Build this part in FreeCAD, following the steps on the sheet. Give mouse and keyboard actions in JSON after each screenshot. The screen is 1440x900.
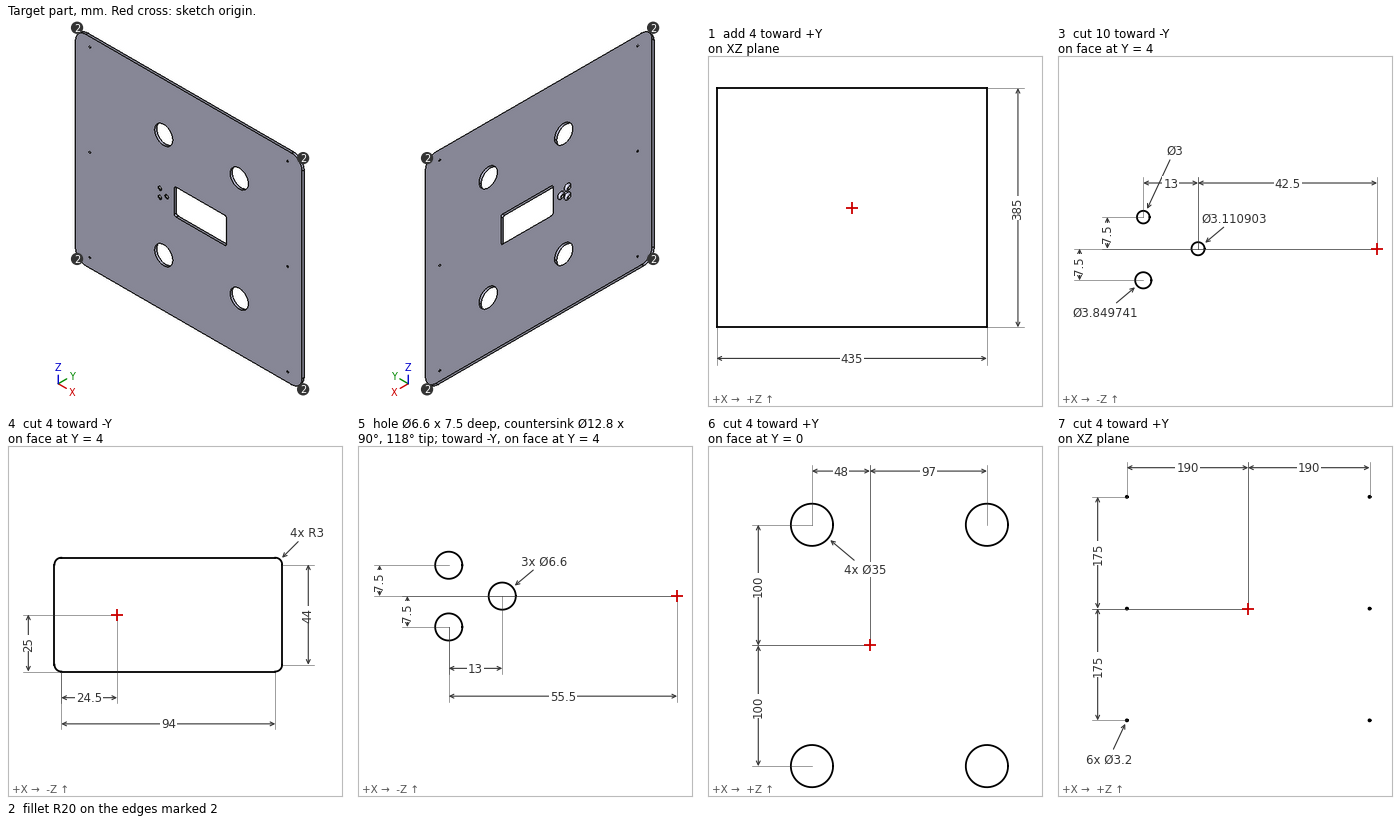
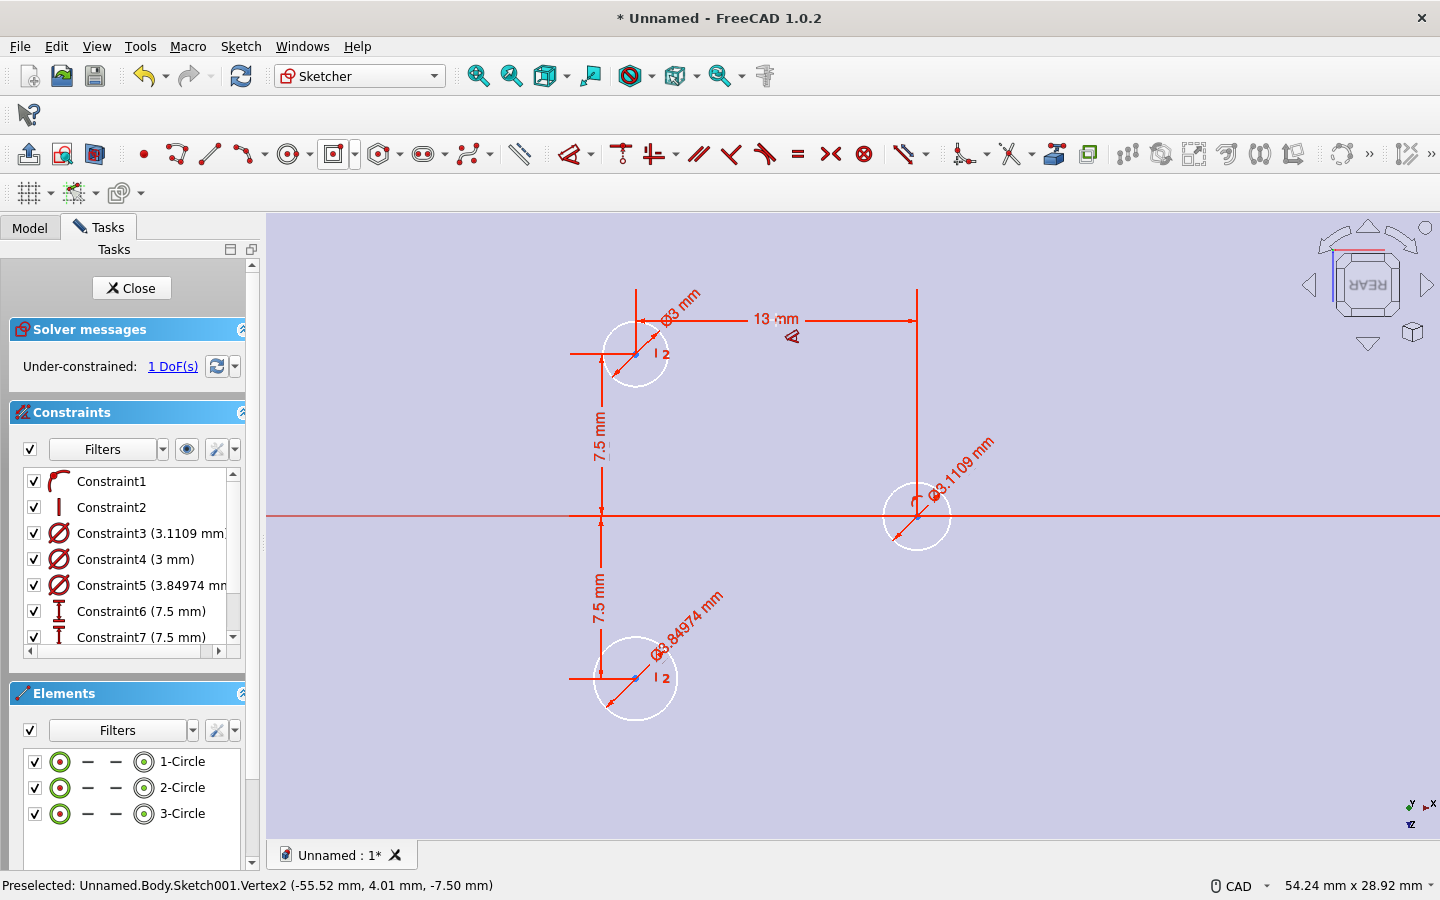
{"action": "left_click", "coordinate": [917, 516]}
{"action": "left_click", "coordinate": [1096, 482]}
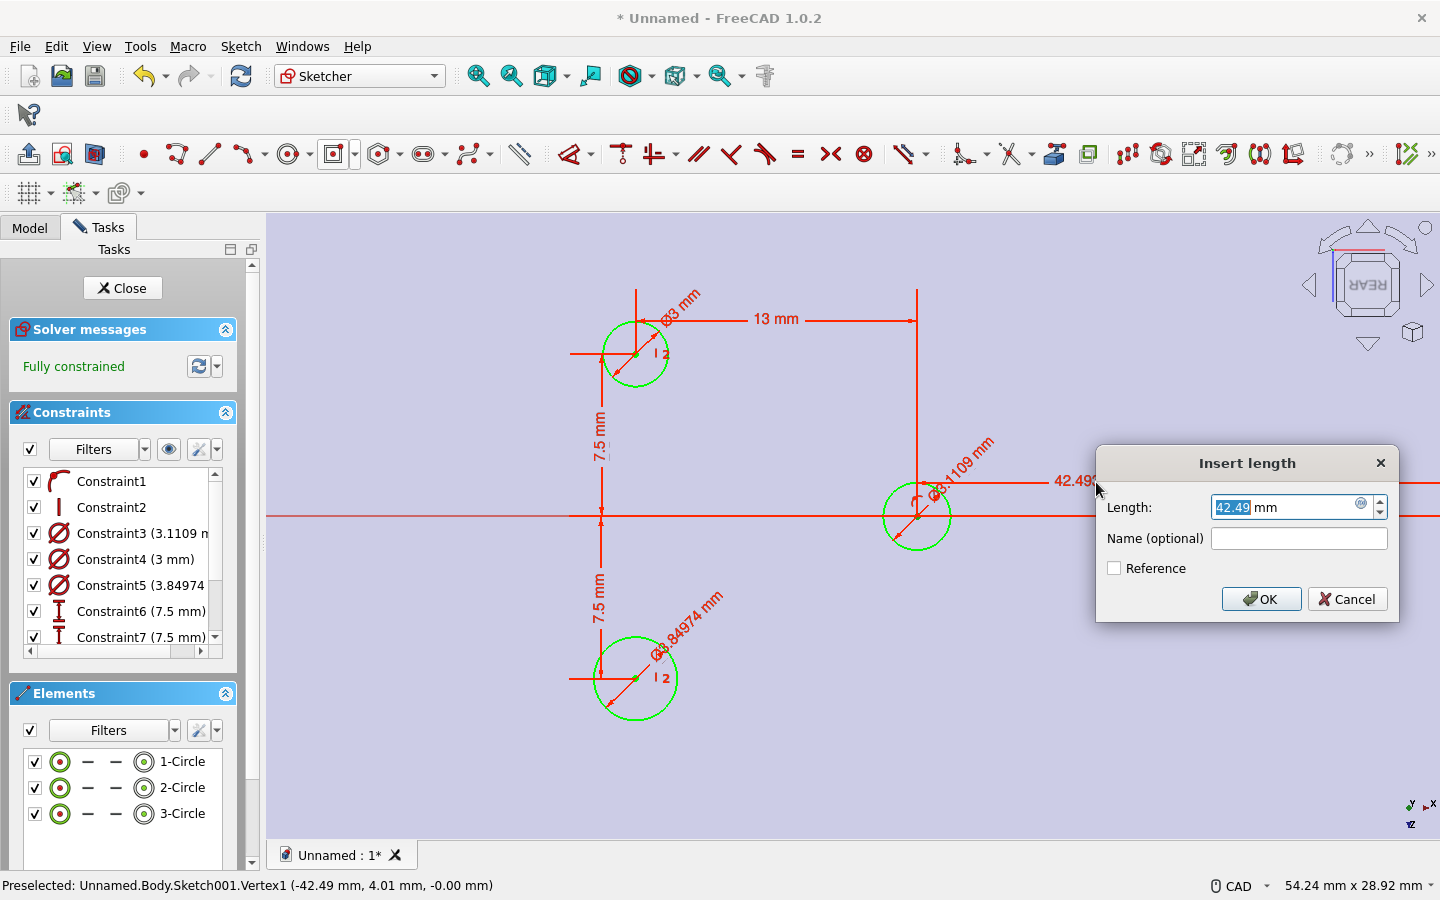
{"action": "type", "text": "42.5"}
{"action": "key", "text": "Return"}
{"action": "key", "text": "Escape"}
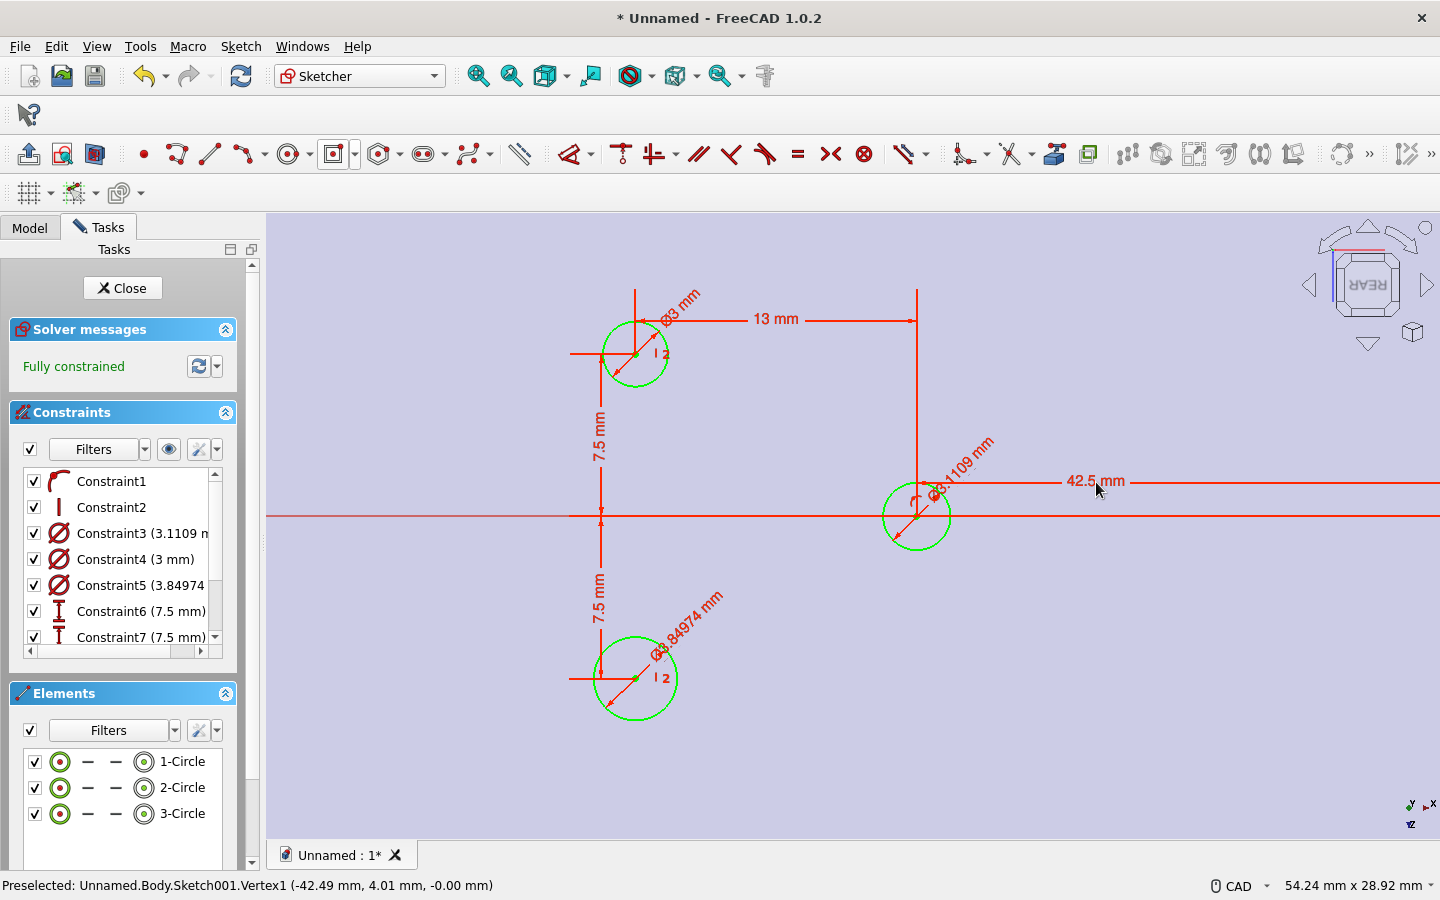
{"action": "left_click", "coordinate": [123, 288]}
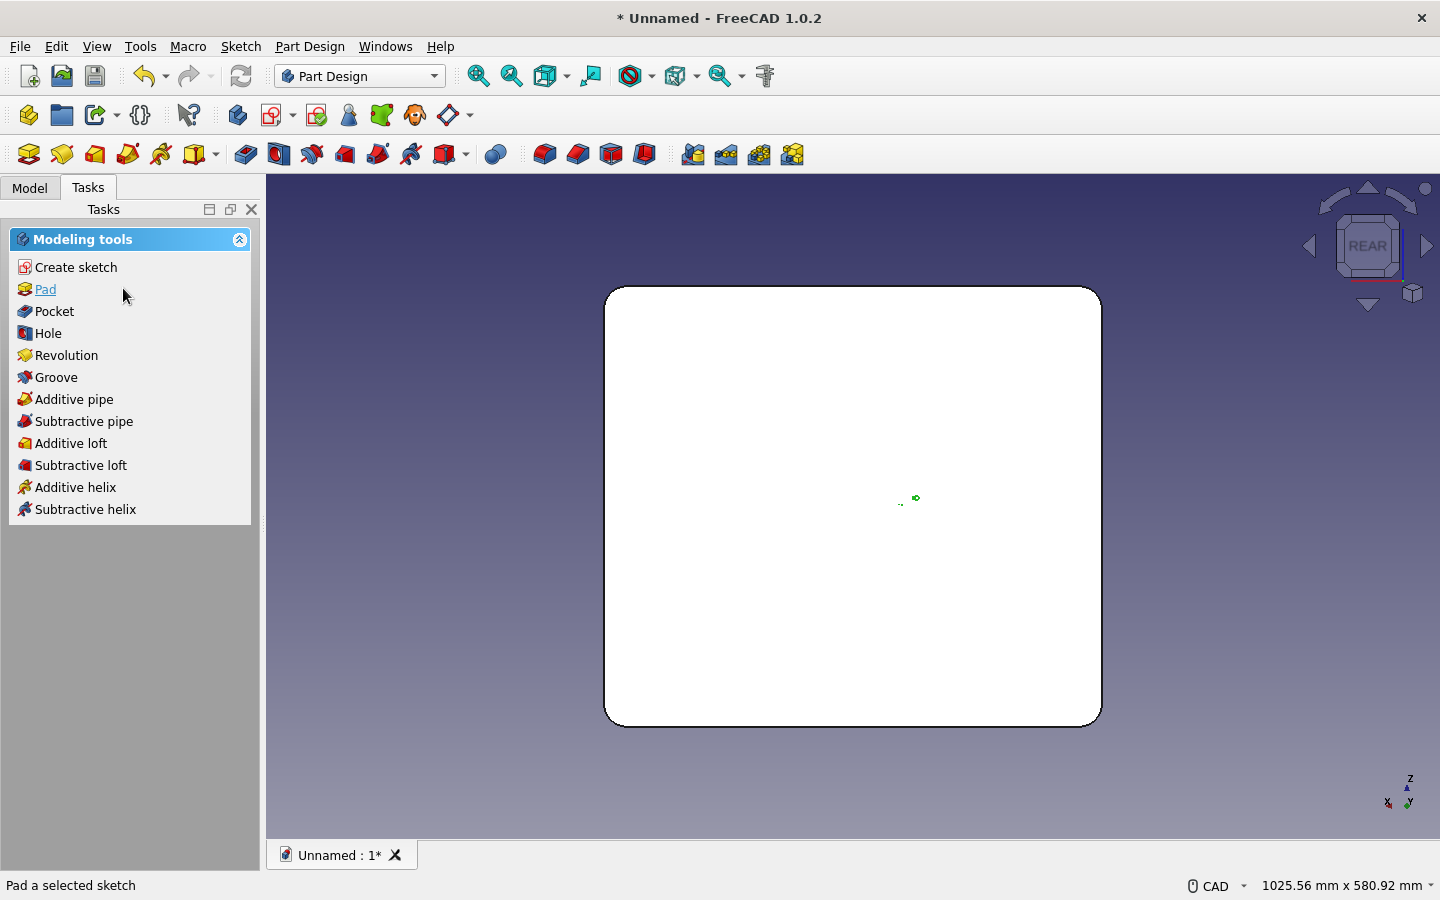
{"action": "left_click", "coordinate": [246, 154]}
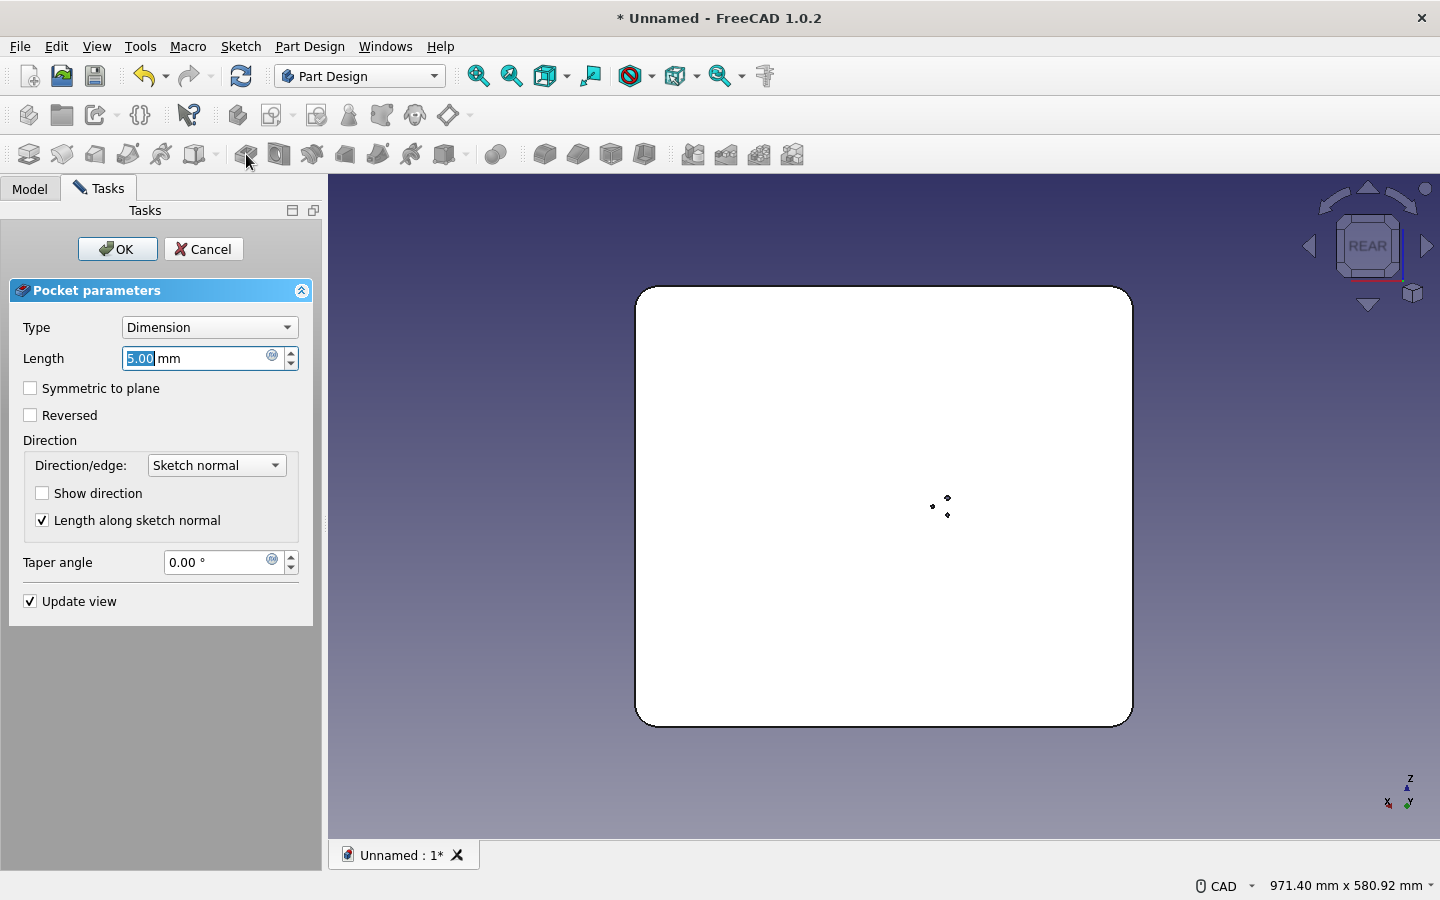
{"action": "type", "text": "10"}
{"action": "key", "text": "Tab"}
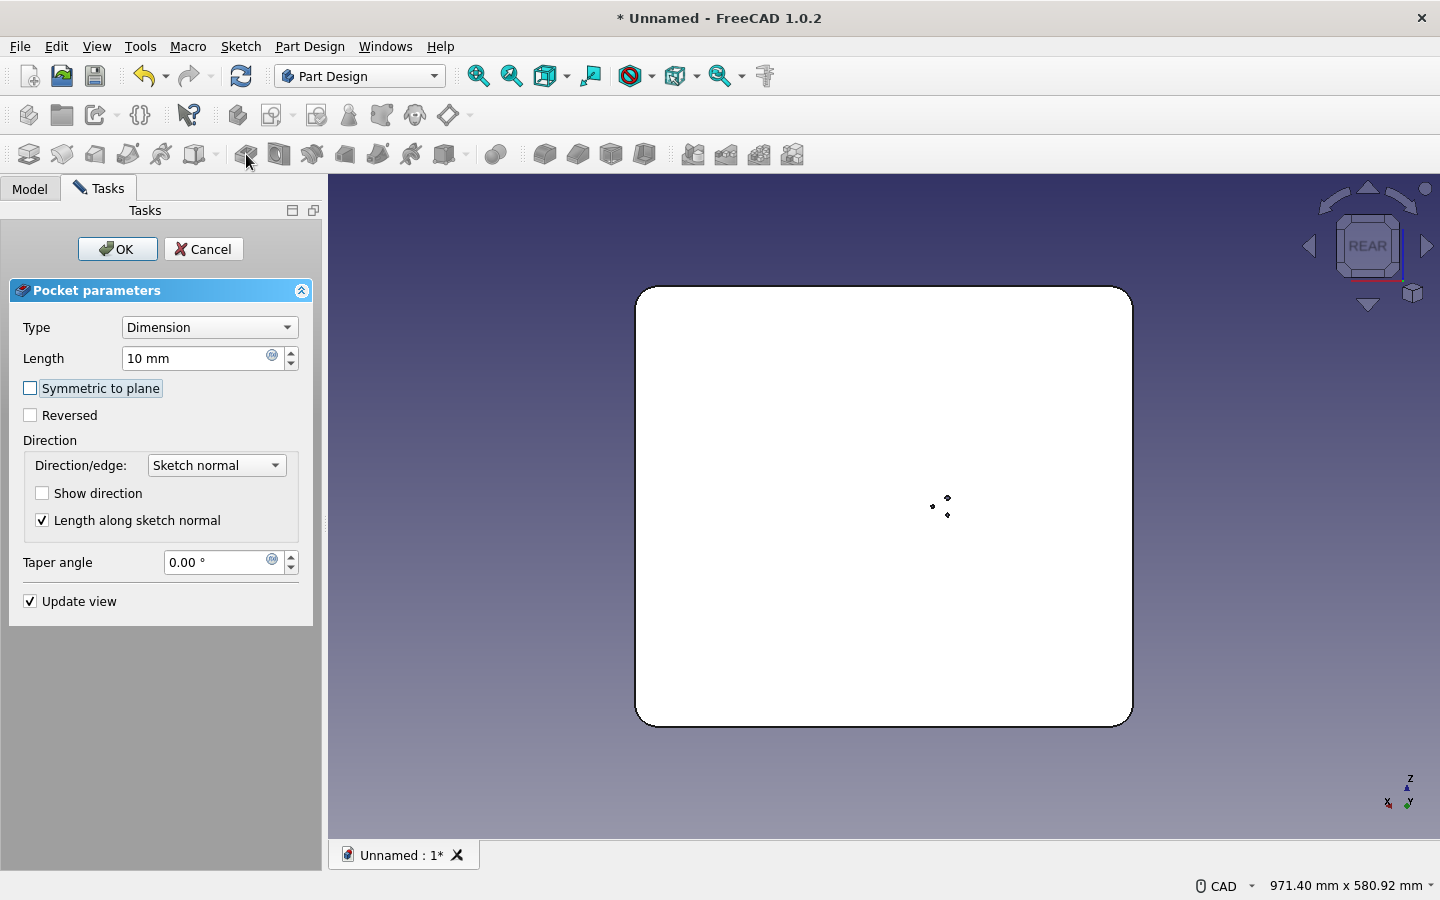
{"action": "left_click", "coordinate": [118, 249]}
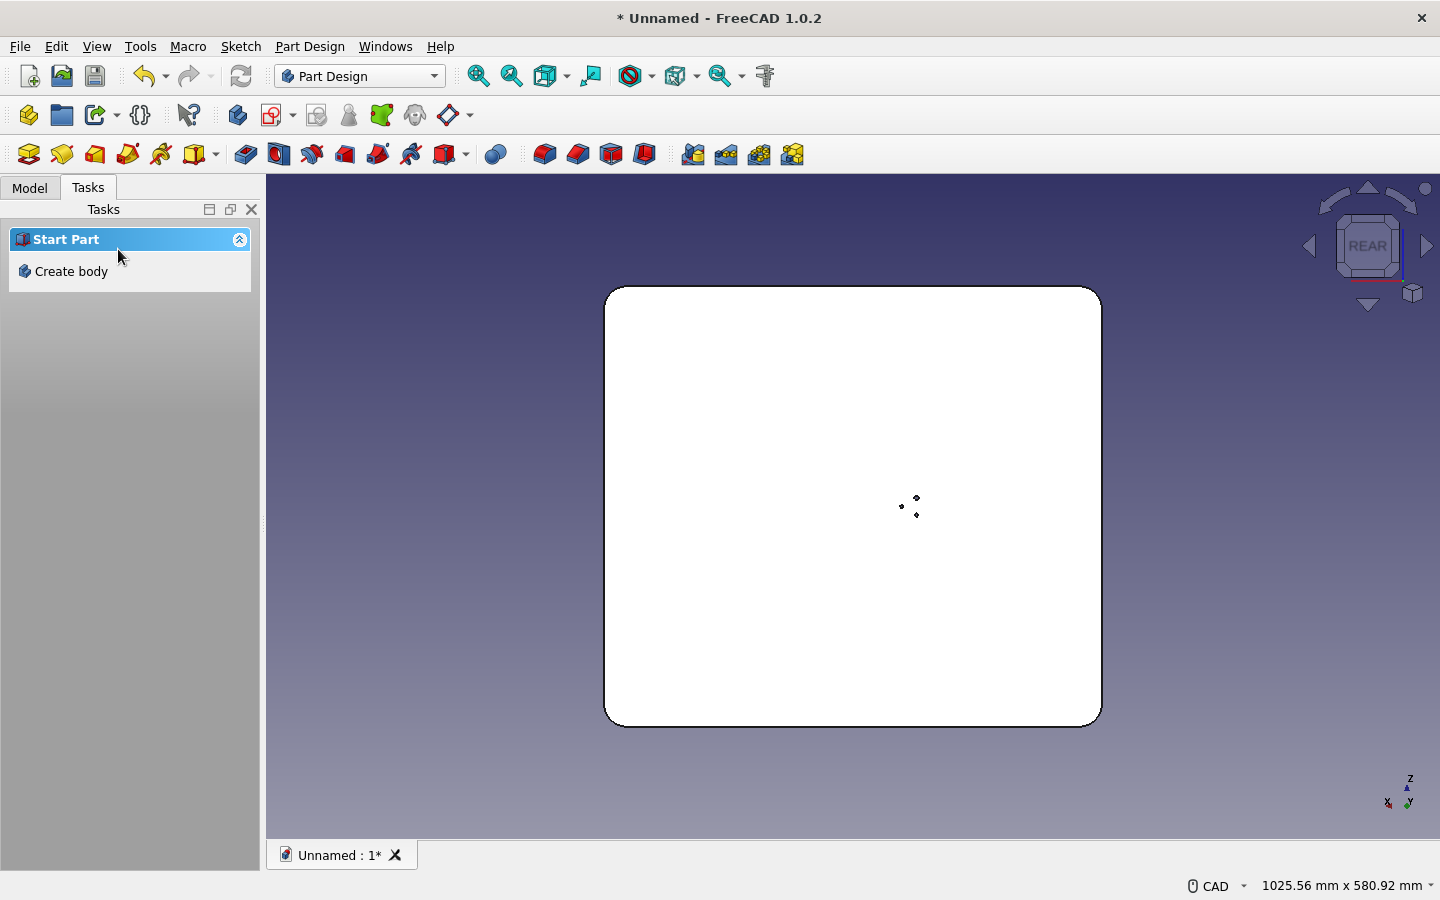
{"action": "left_click", "coordinate": [782, 443]}